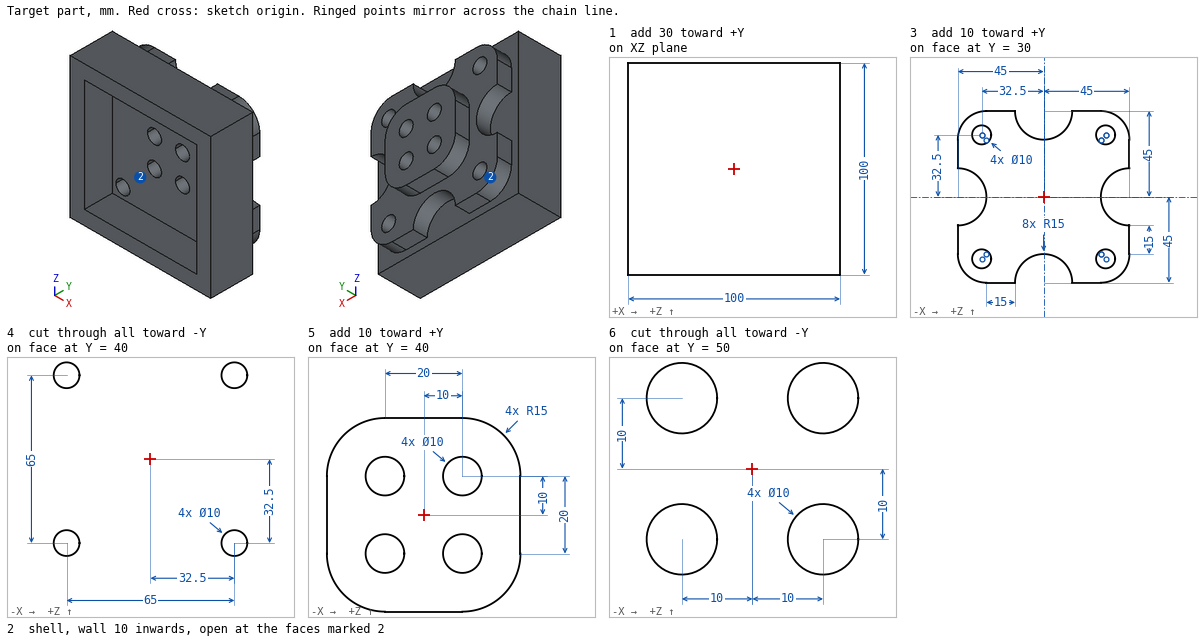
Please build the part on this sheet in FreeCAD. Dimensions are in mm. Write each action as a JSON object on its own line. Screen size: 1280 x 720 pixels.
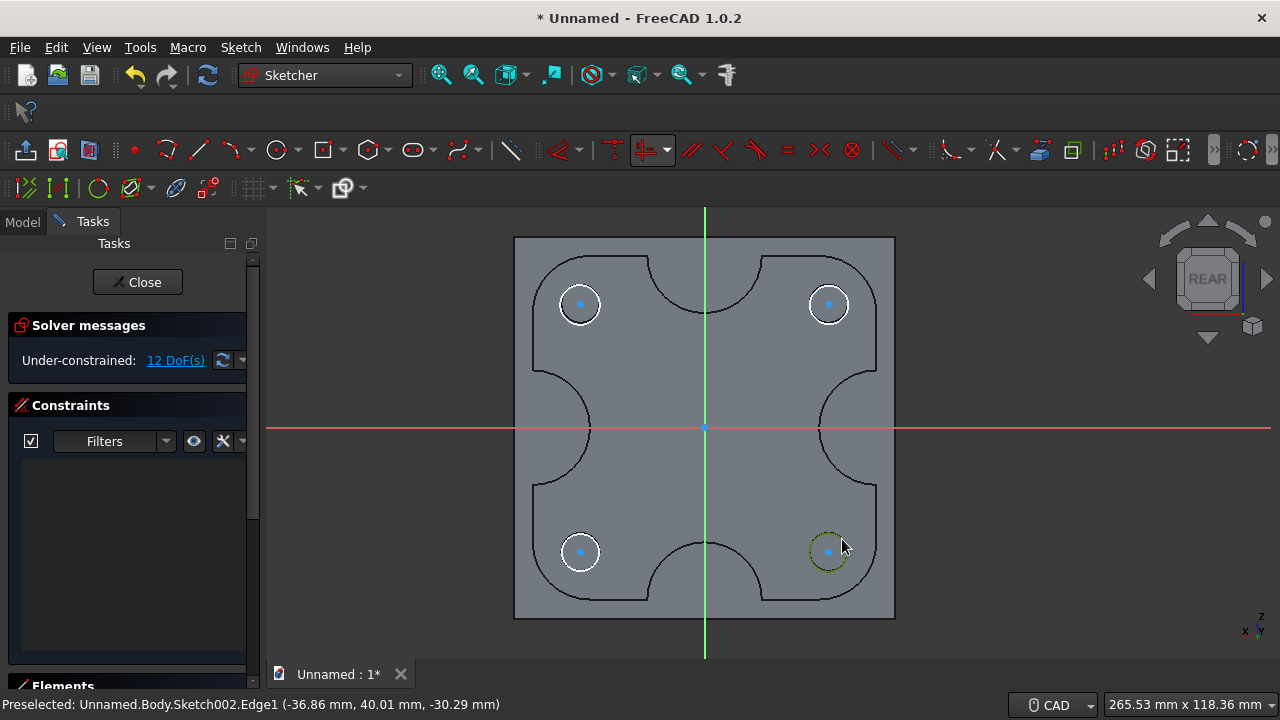
{"action": "left_click", "coordinate": [594, 539]}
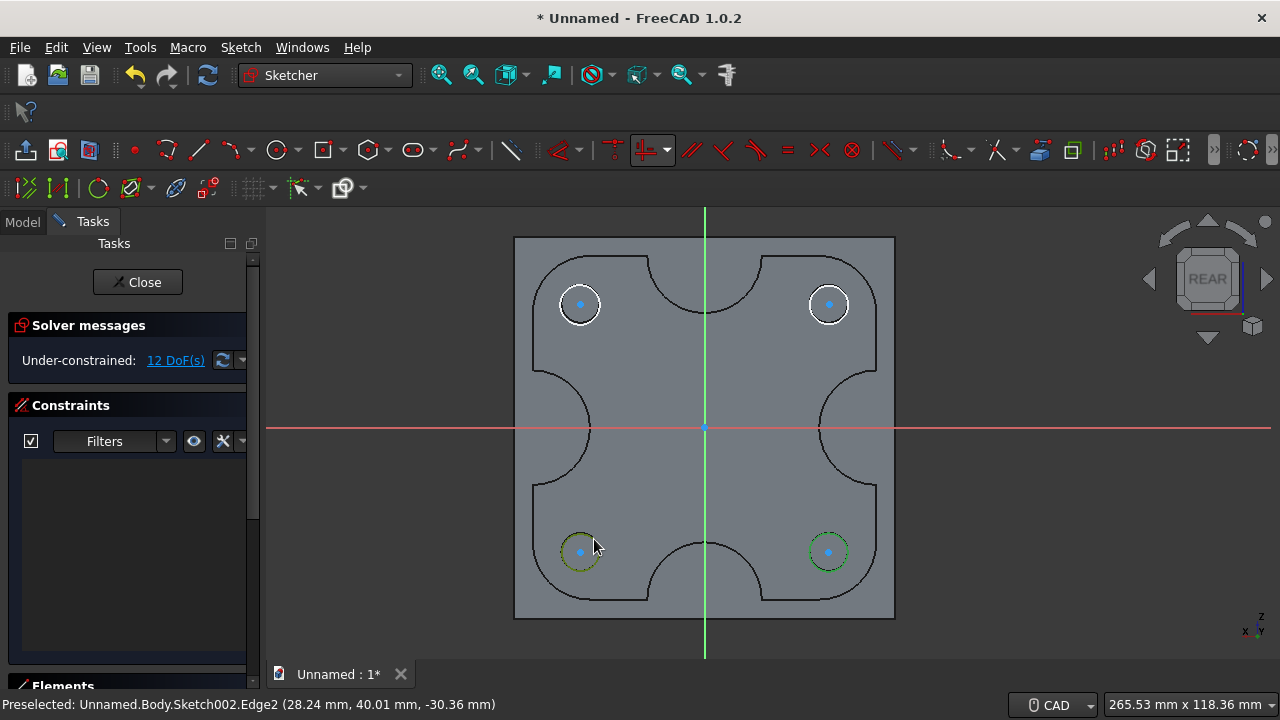
{"action": "left_click", "coordinate": [594, 291]}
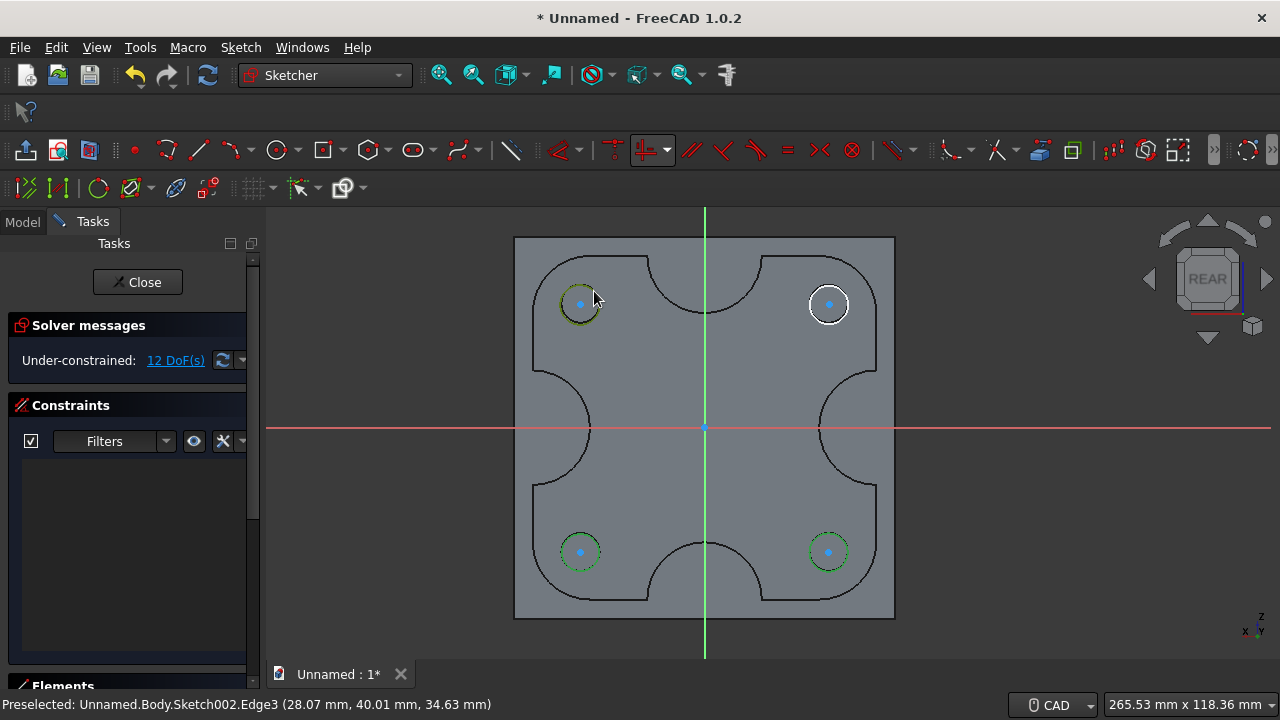
{"action": "left_click", "coordinate": [842, 291]}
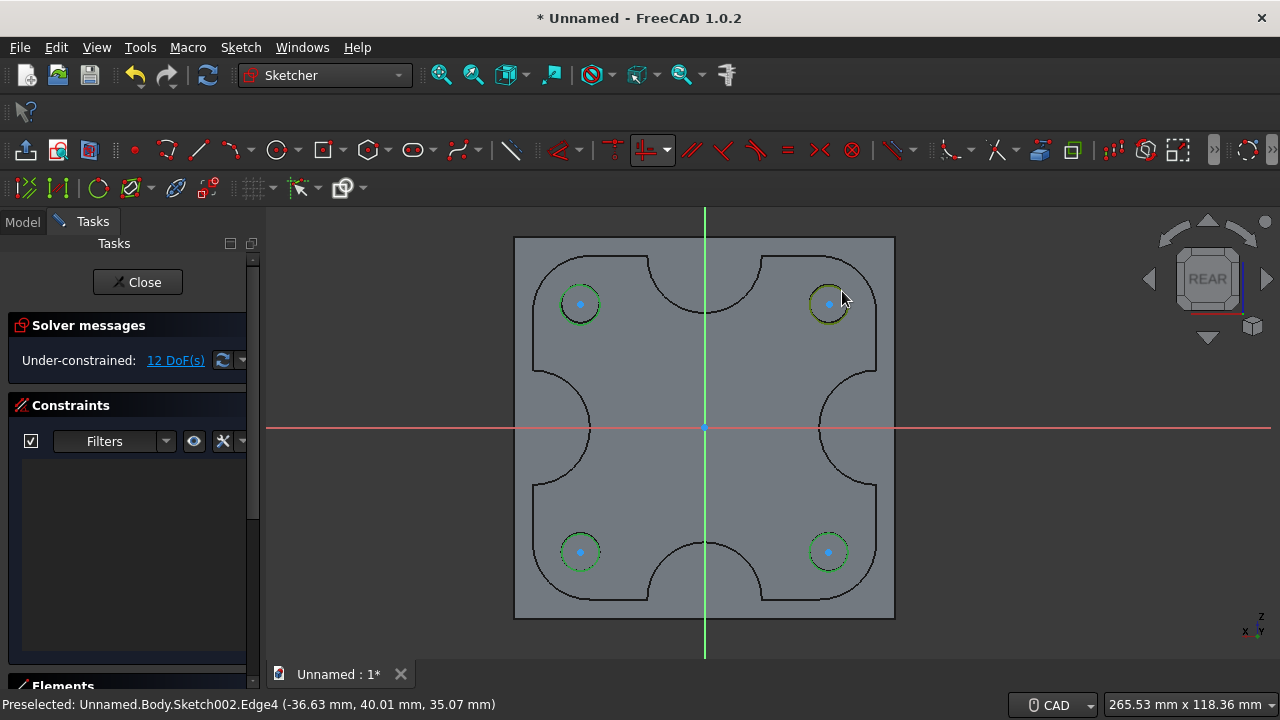
{"action": "left_click", "coordinate": [788, 150]}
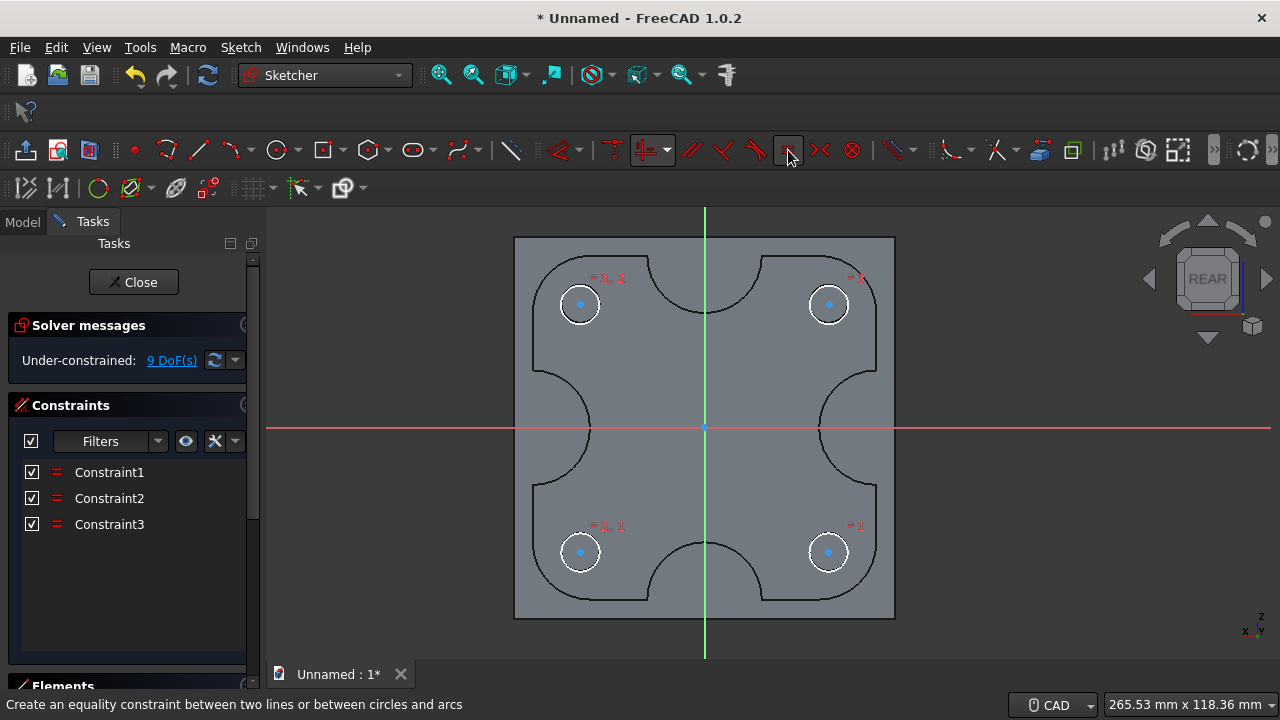
{"action": "left_click", "coordinate": [829, 553]}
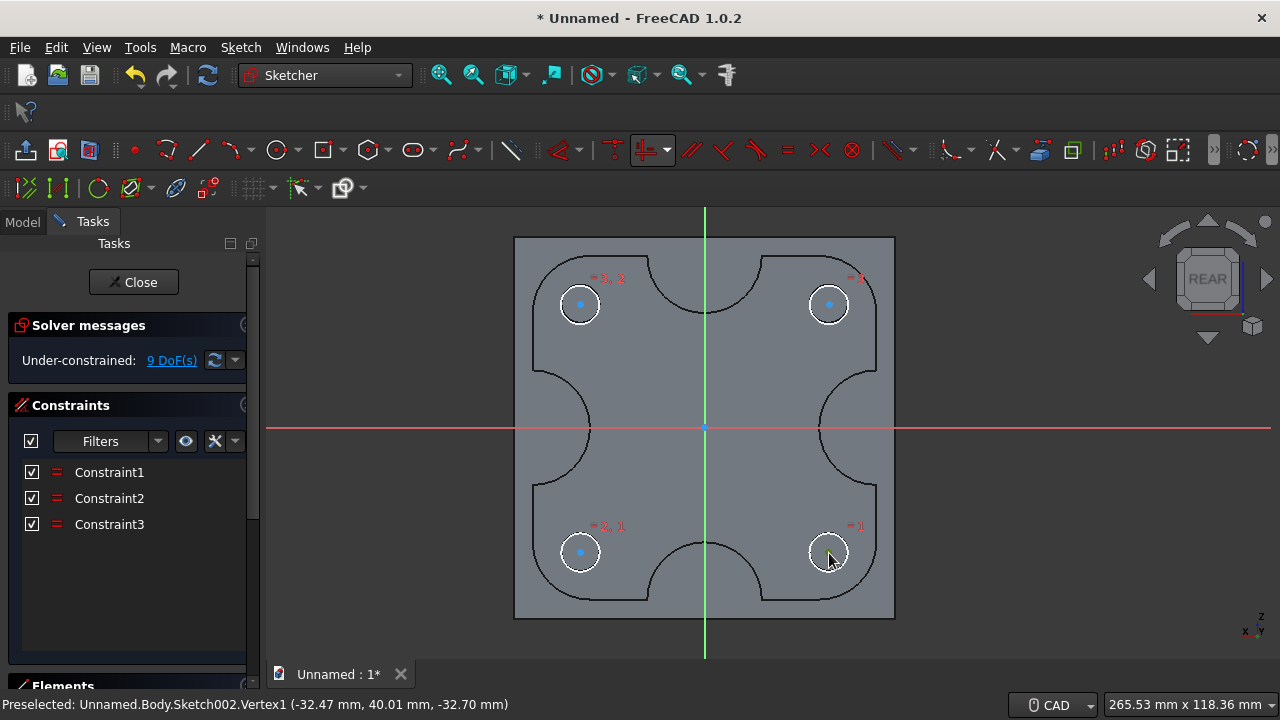
{"action": "left_click", "coordinate": [580, 553]}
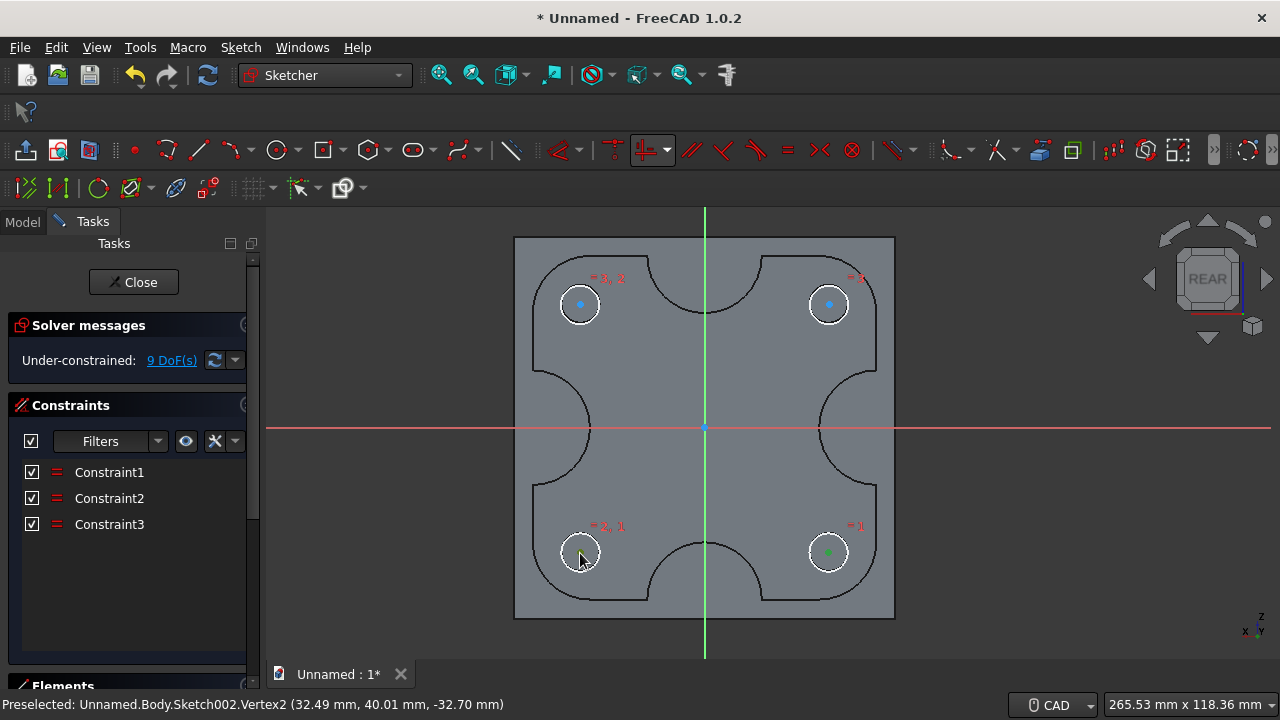
{"action": "left_click", "coordinate": [670, 150]}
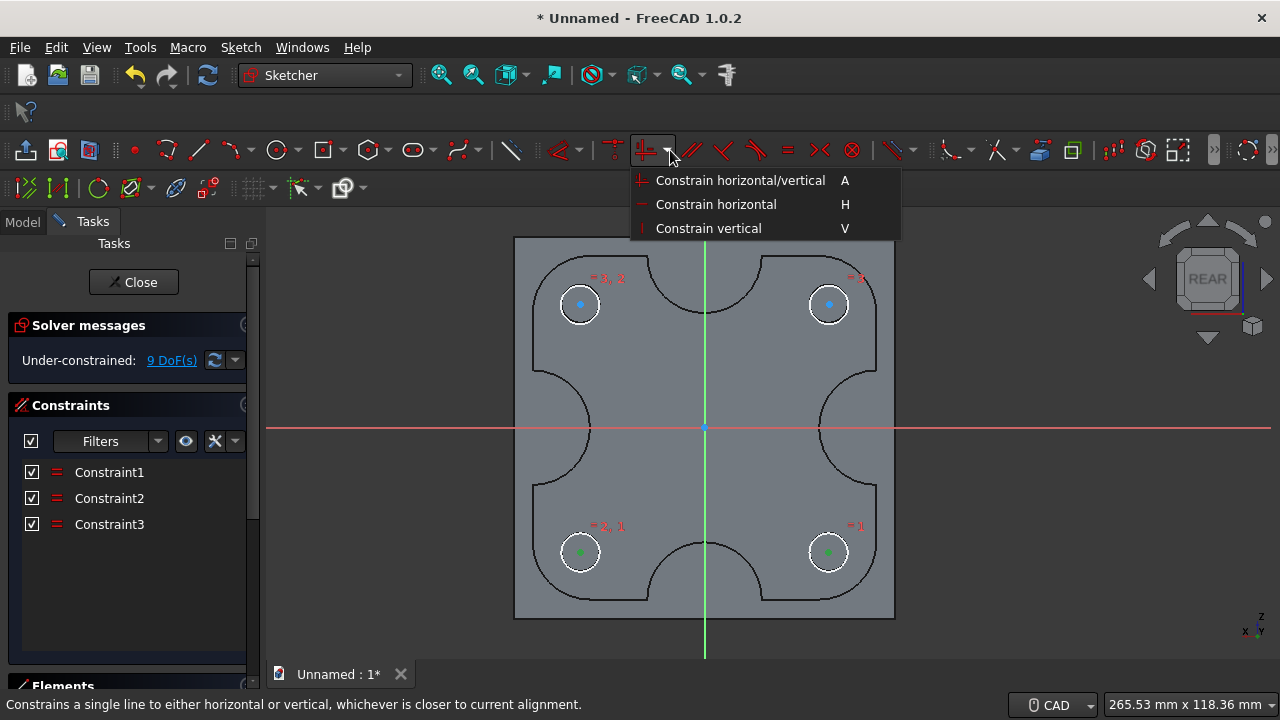
{"action": "left_click", "coordinate": [766, 204]}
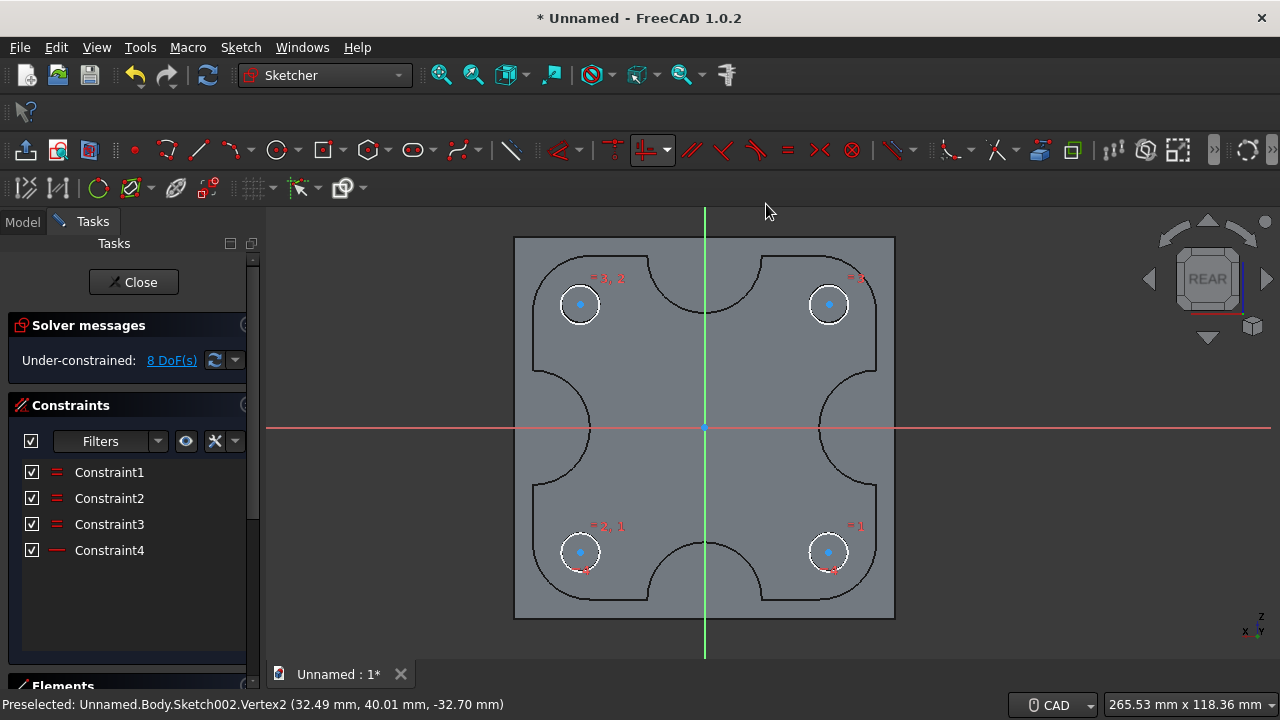
{"action": "left_click", "coordinate": [580, 553]}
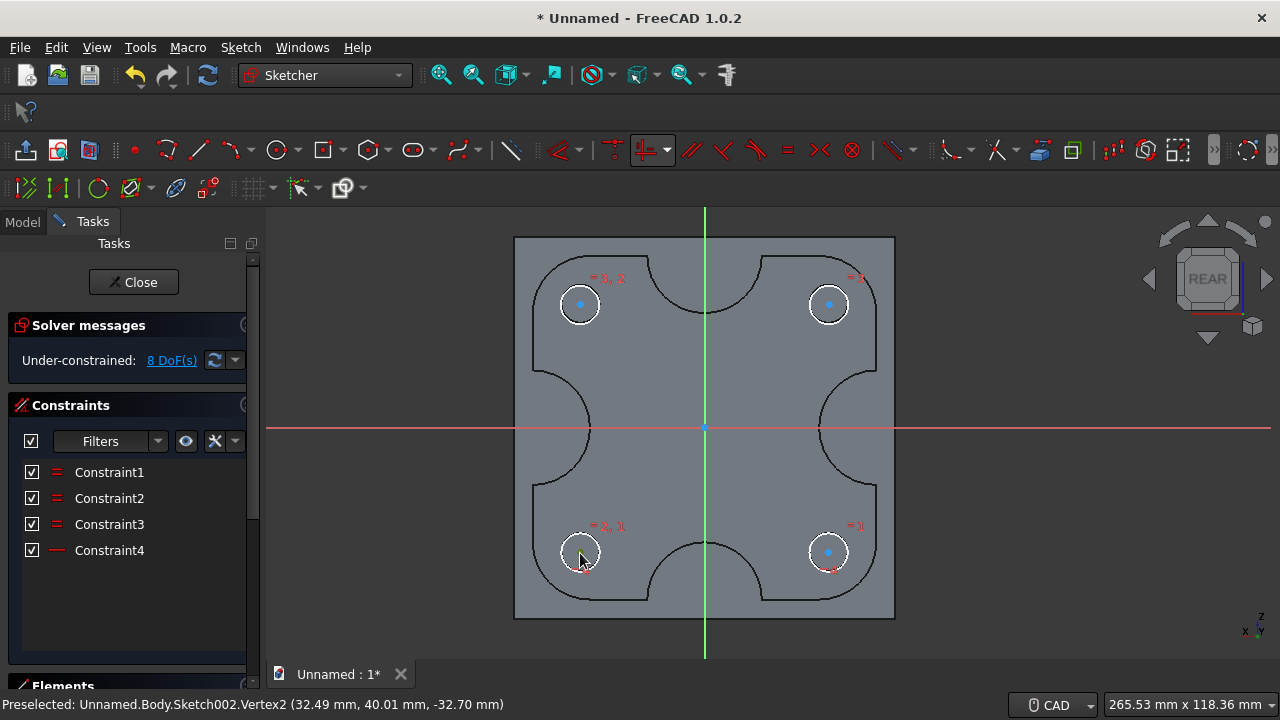
{"action": "left_click", "coordinate": [580, 305]}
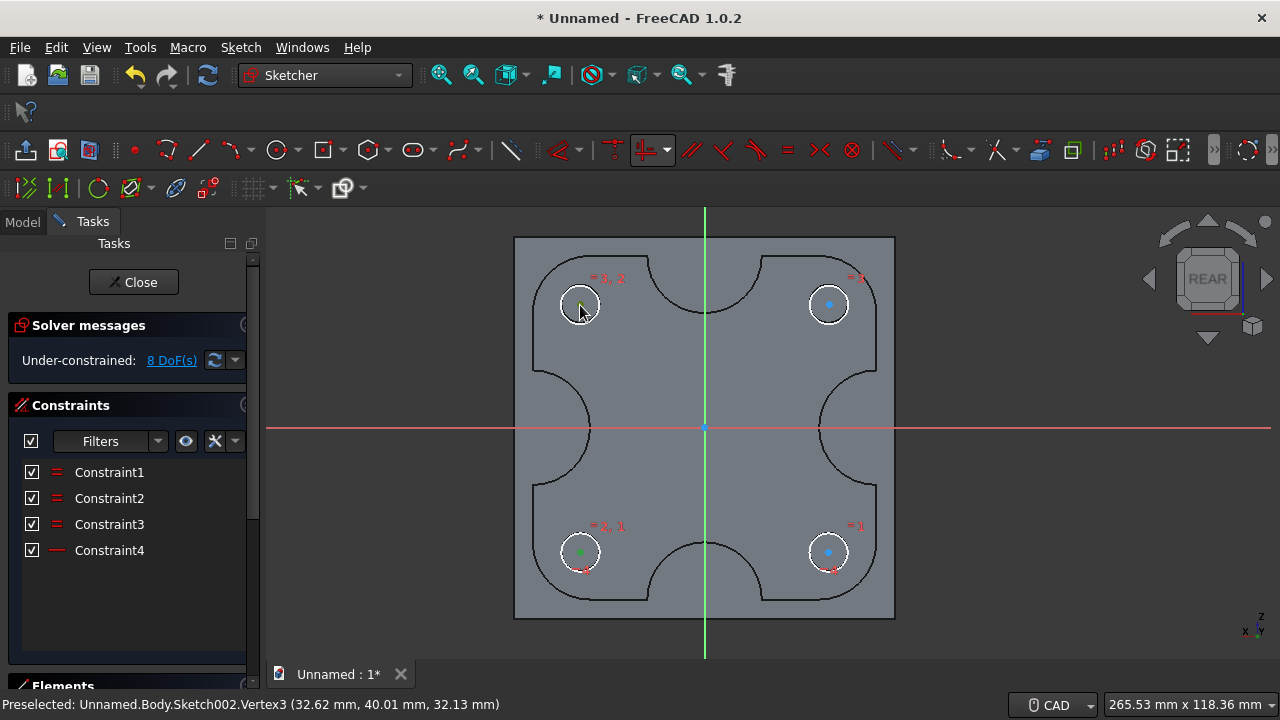
{"action": "key", "text": "v"}